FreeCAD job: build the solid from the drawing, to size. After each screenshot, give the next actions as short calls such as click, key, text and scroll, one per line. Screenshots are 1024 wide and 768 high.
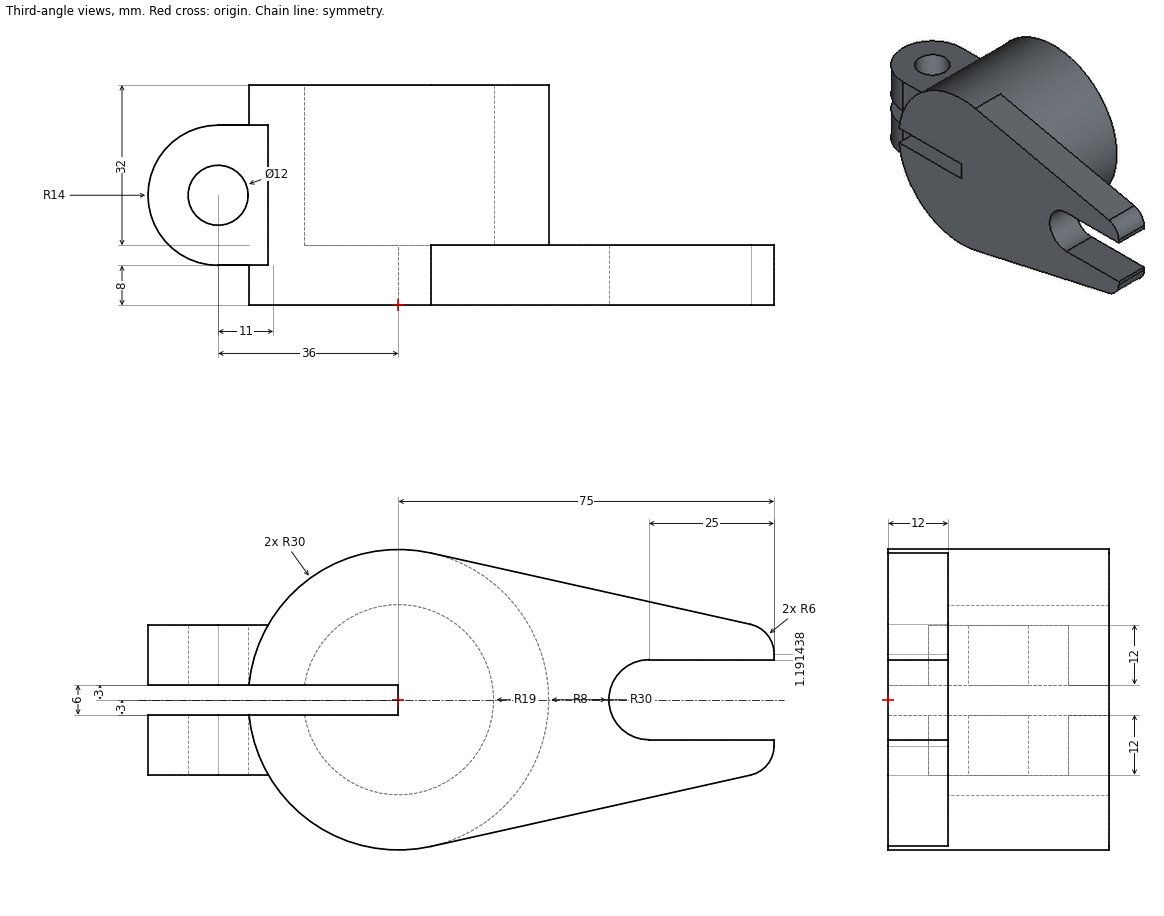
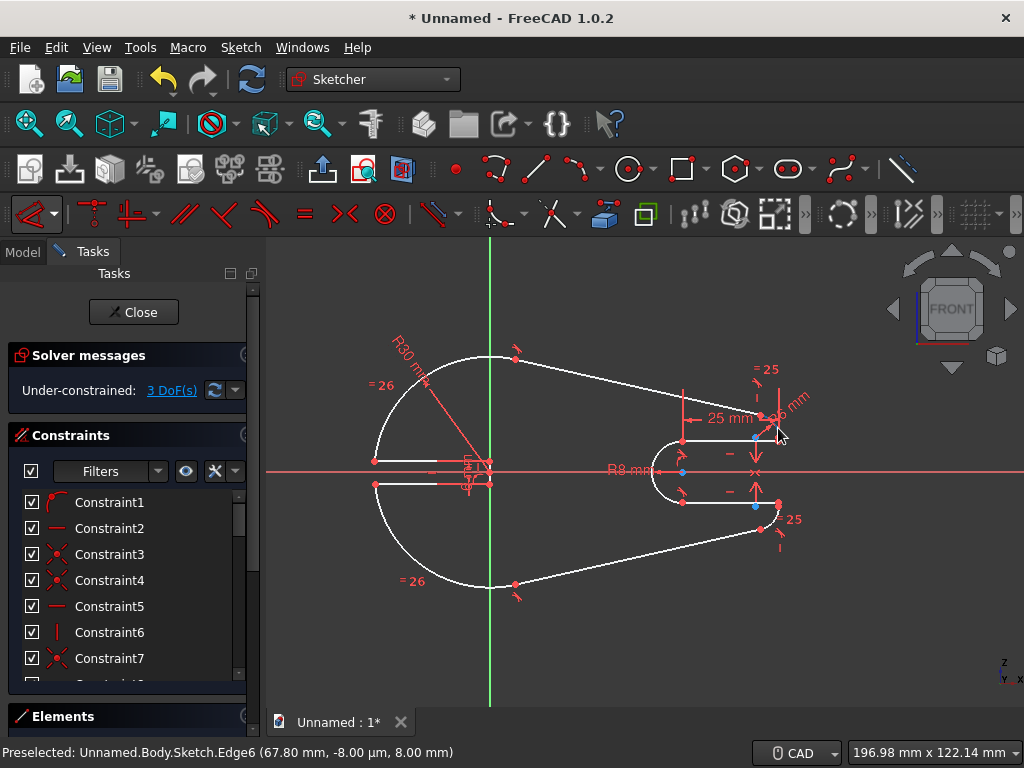
scroll(375, 484, up, 7)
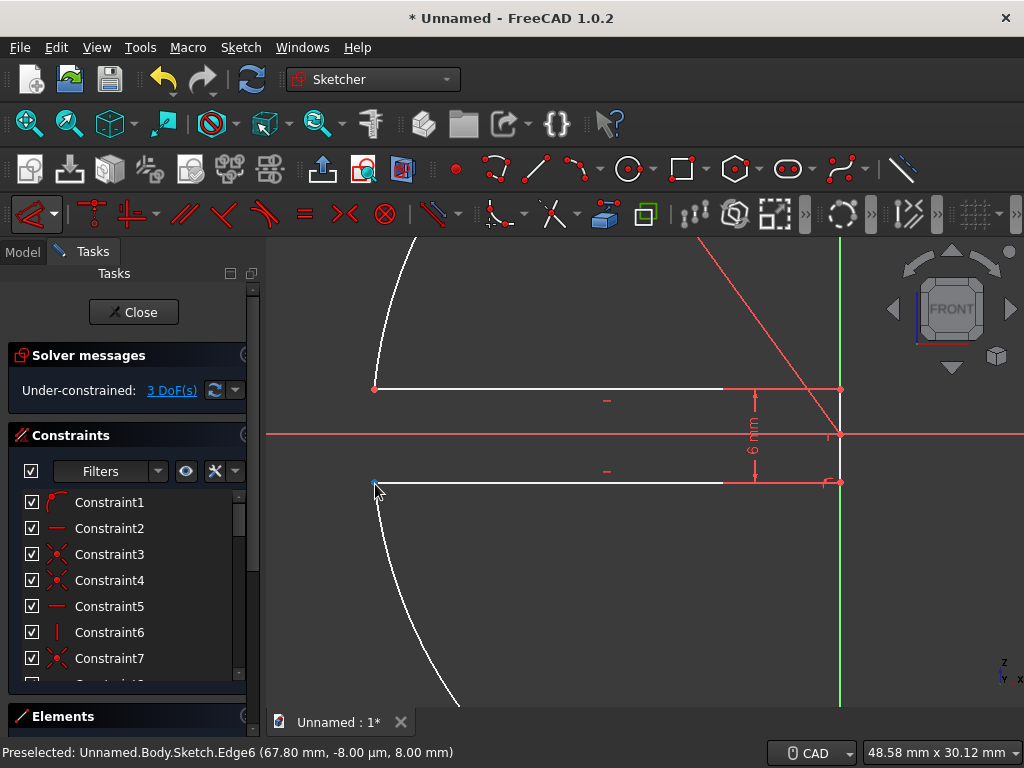
click(375, 483)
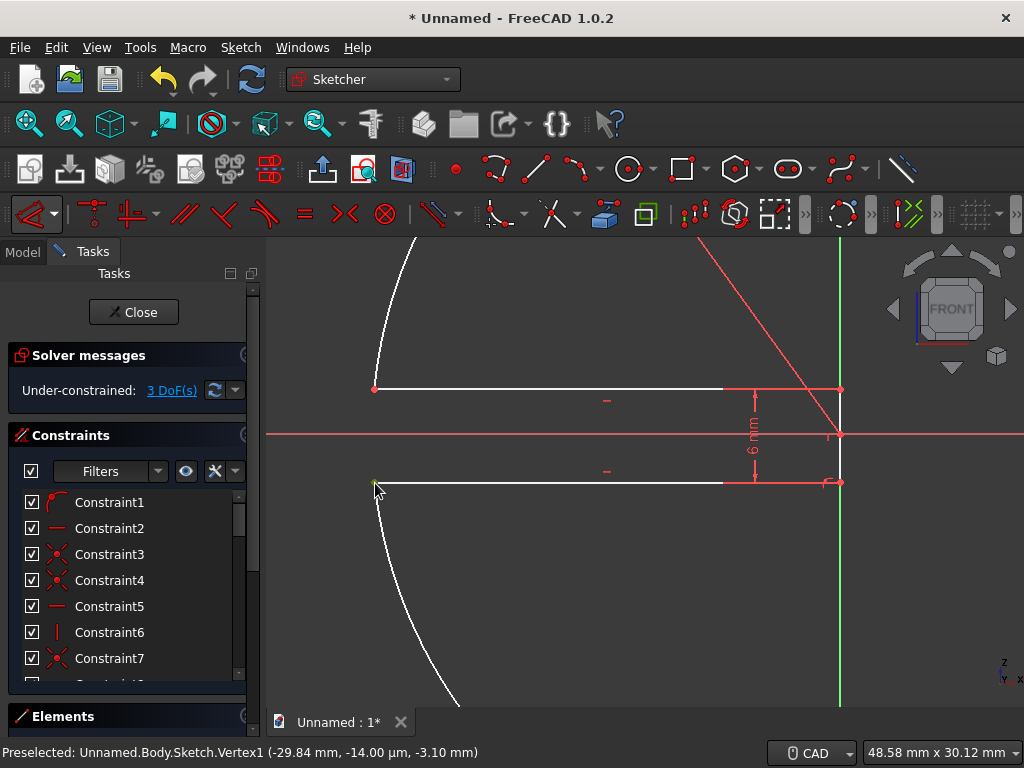
click(56, 214)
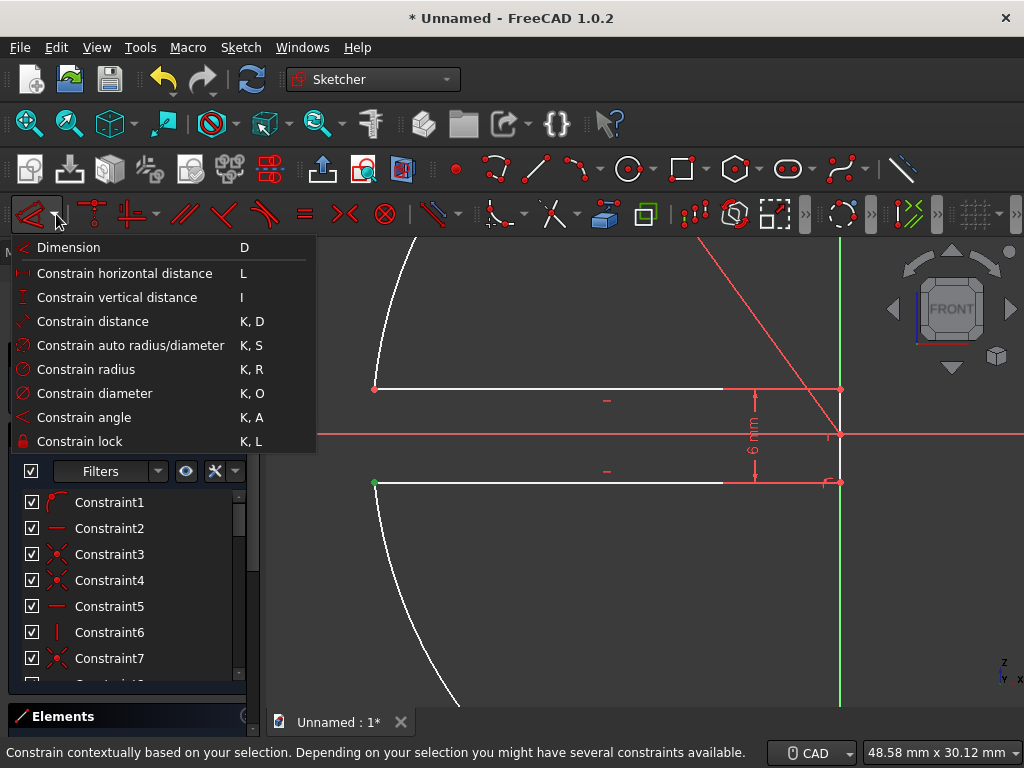
click(164, 297)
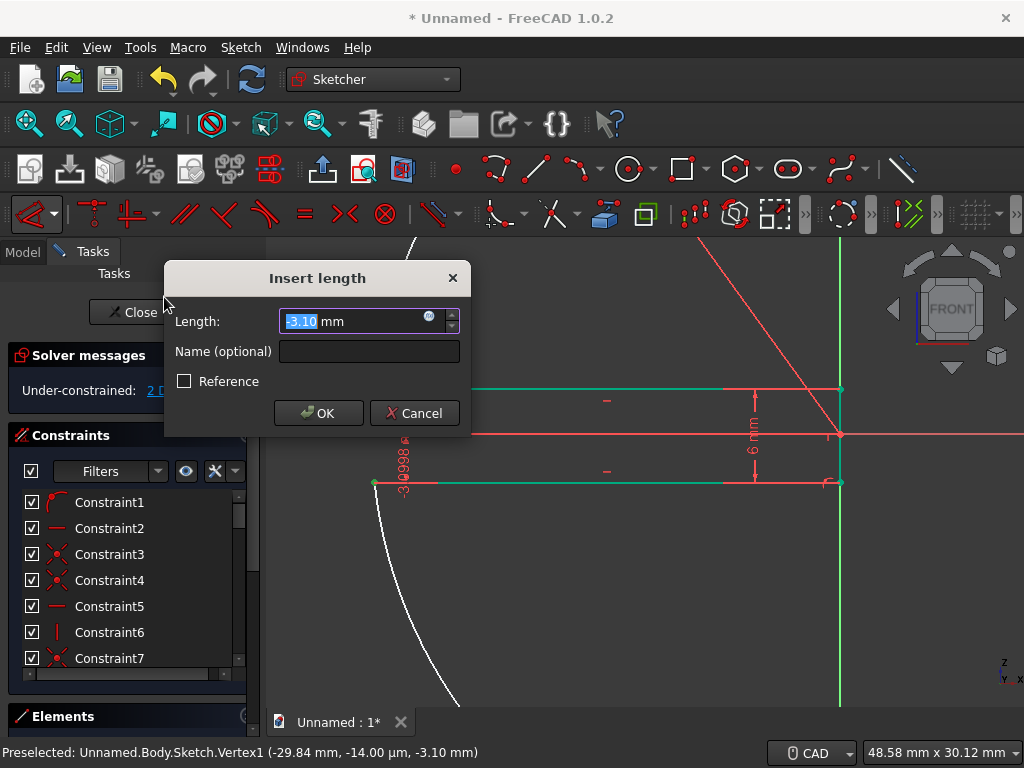
text(-3)
key(Return)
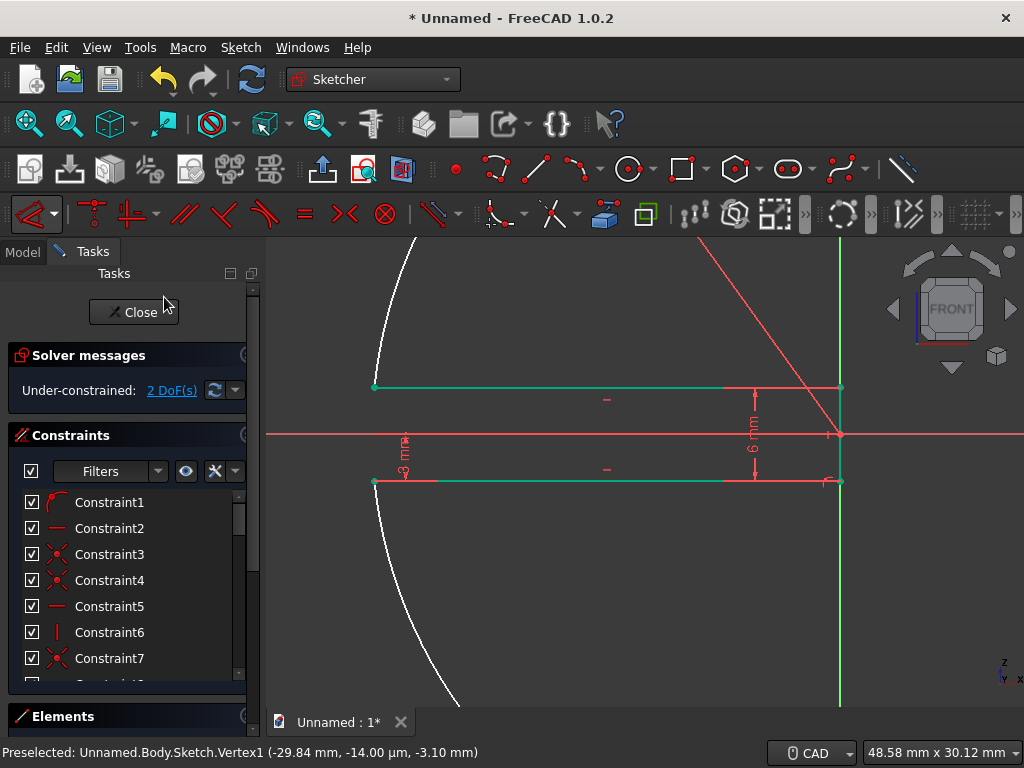
scroll(375, 484, down, 7)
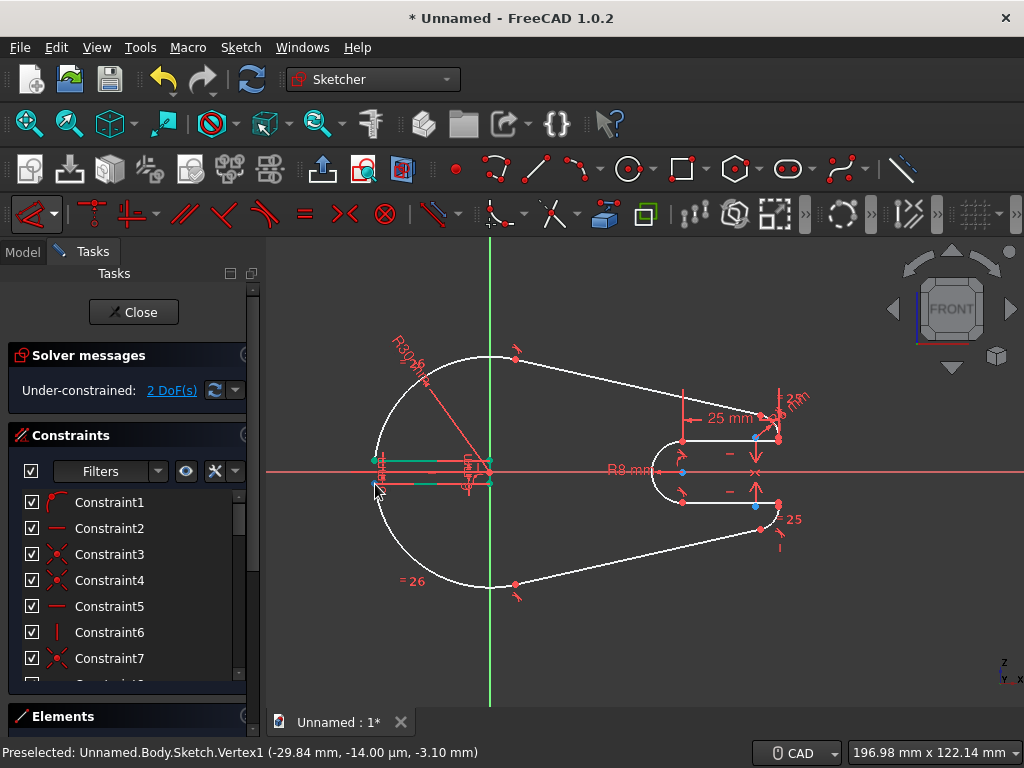
scroll(779, 438, up, 6)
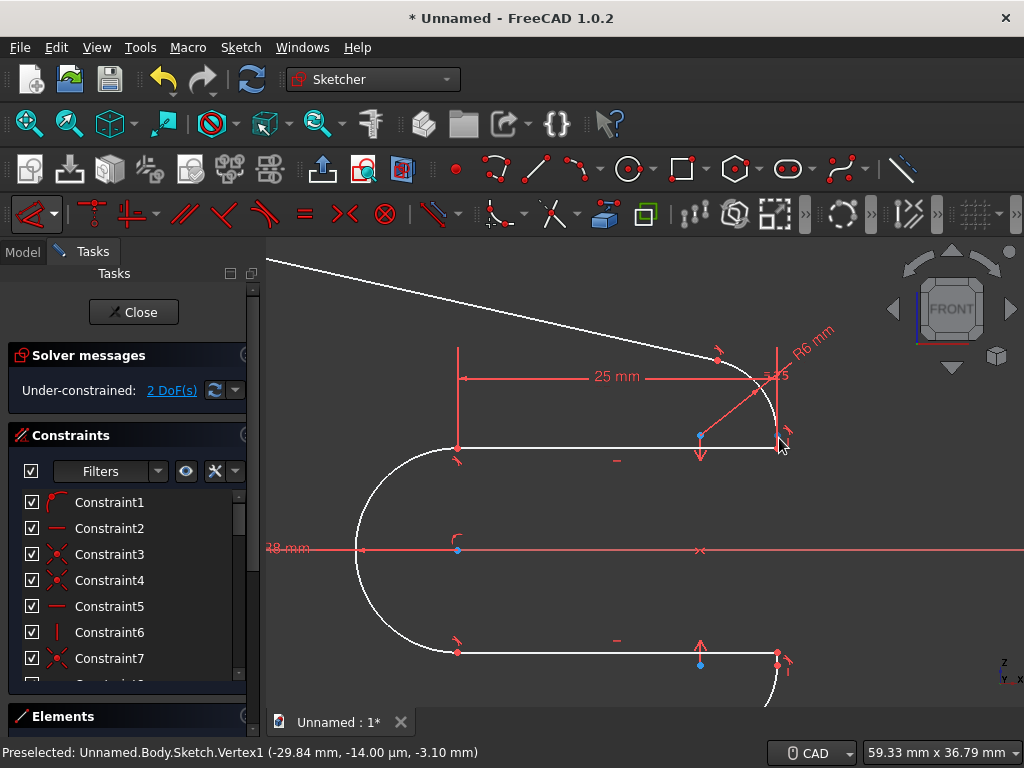
click(777, 435)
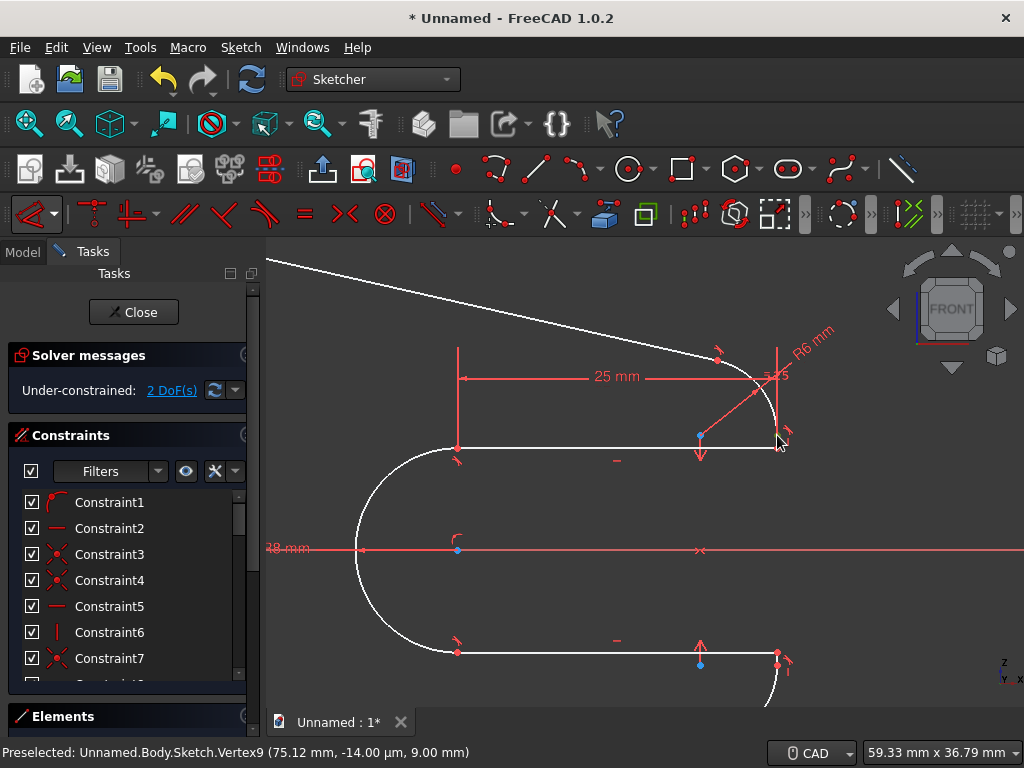
key(l)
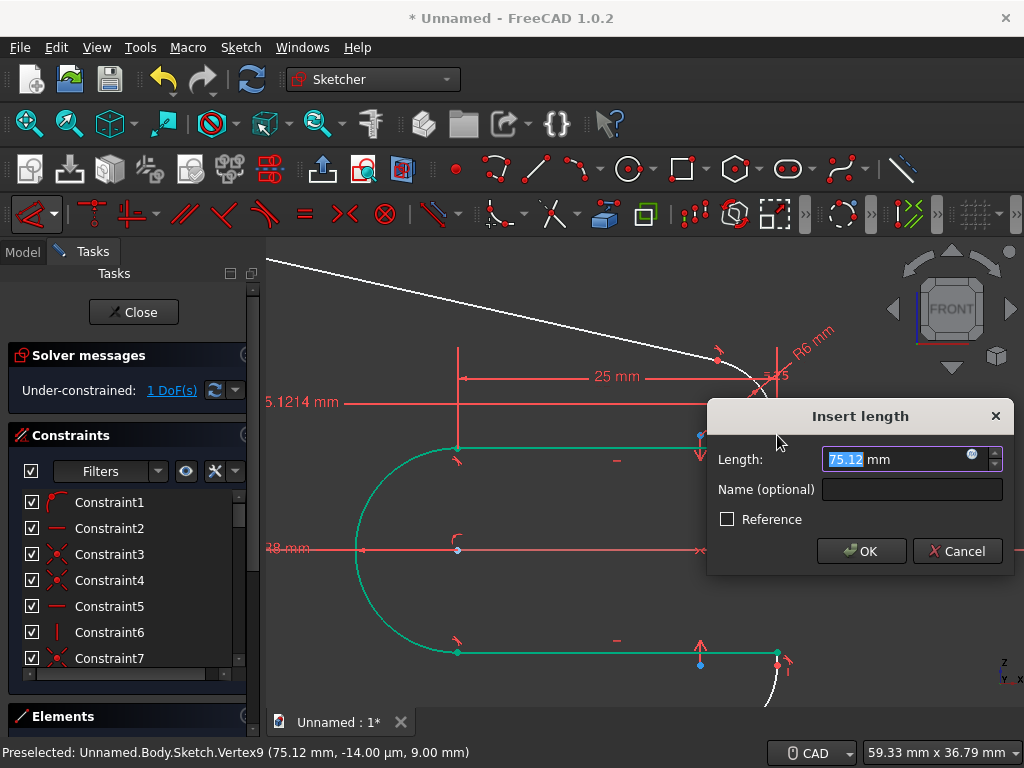
text(75)
key(Return)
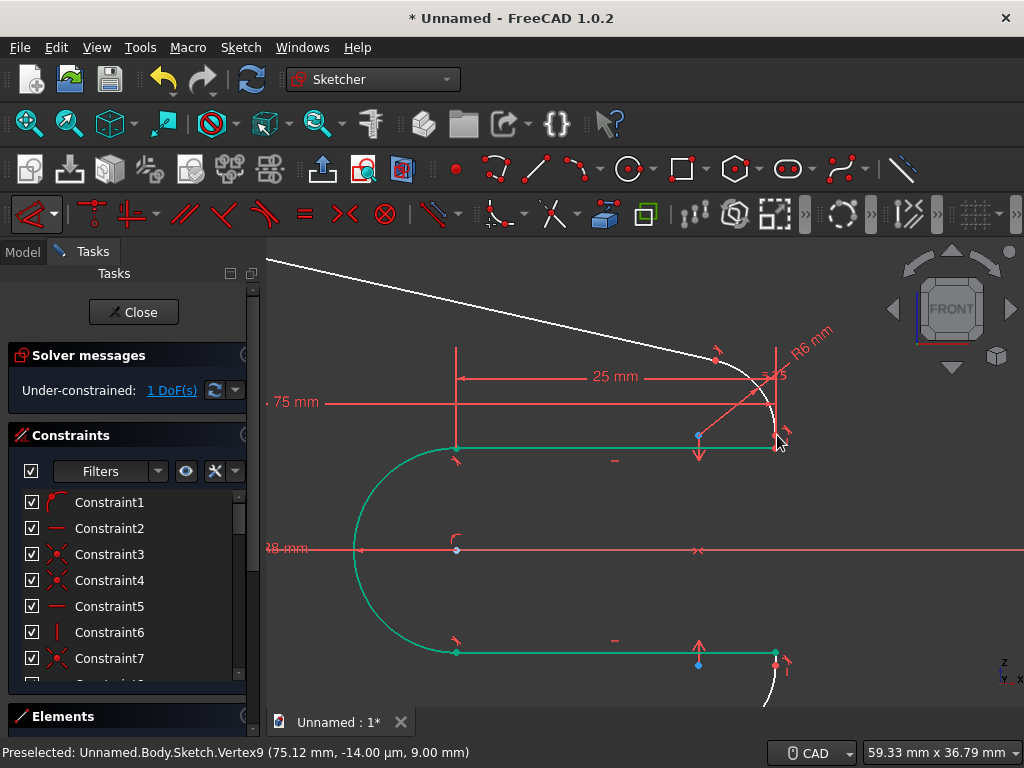
scroll(776, 442, up, 5)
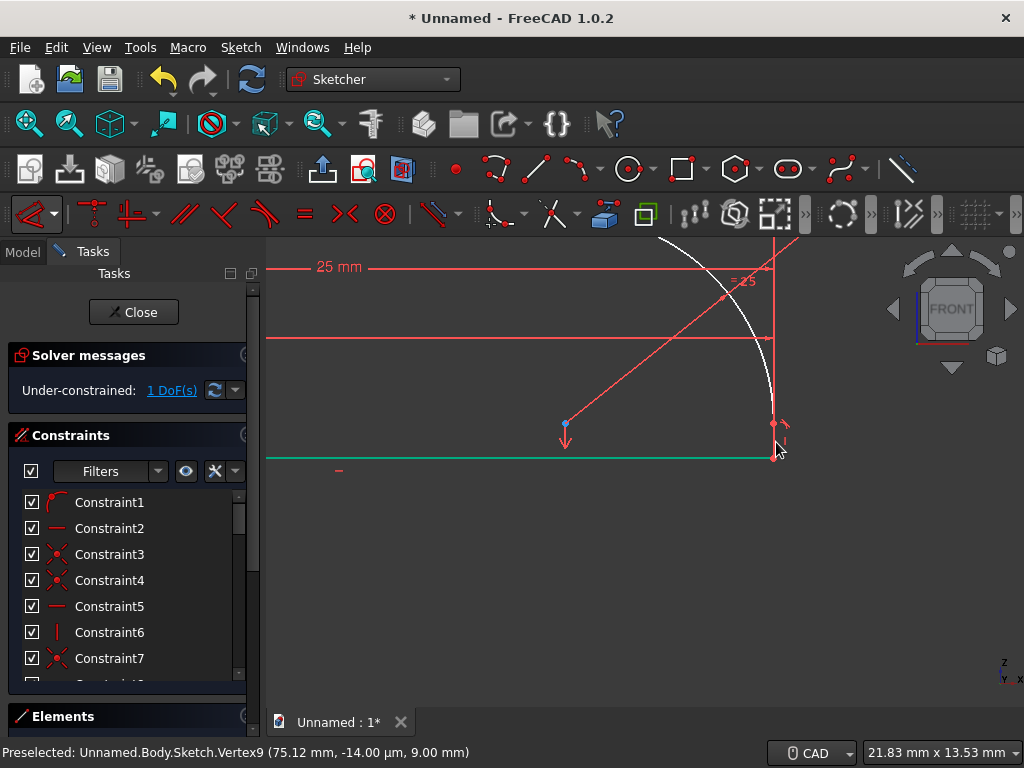
click(774, 441)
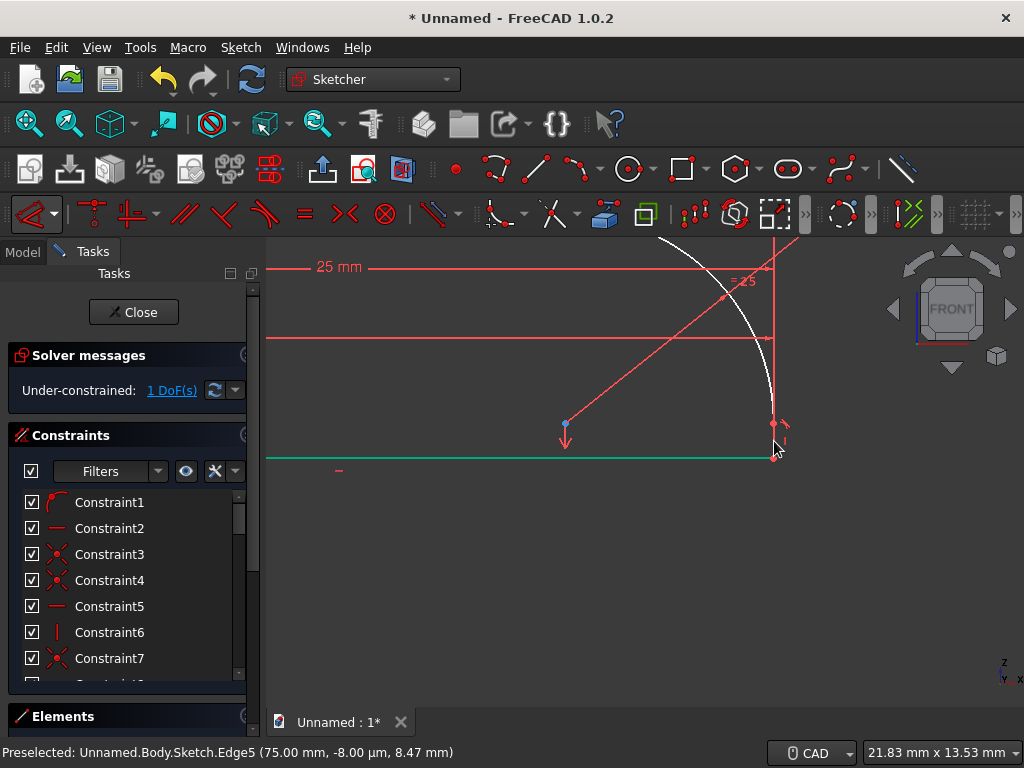
key(i)